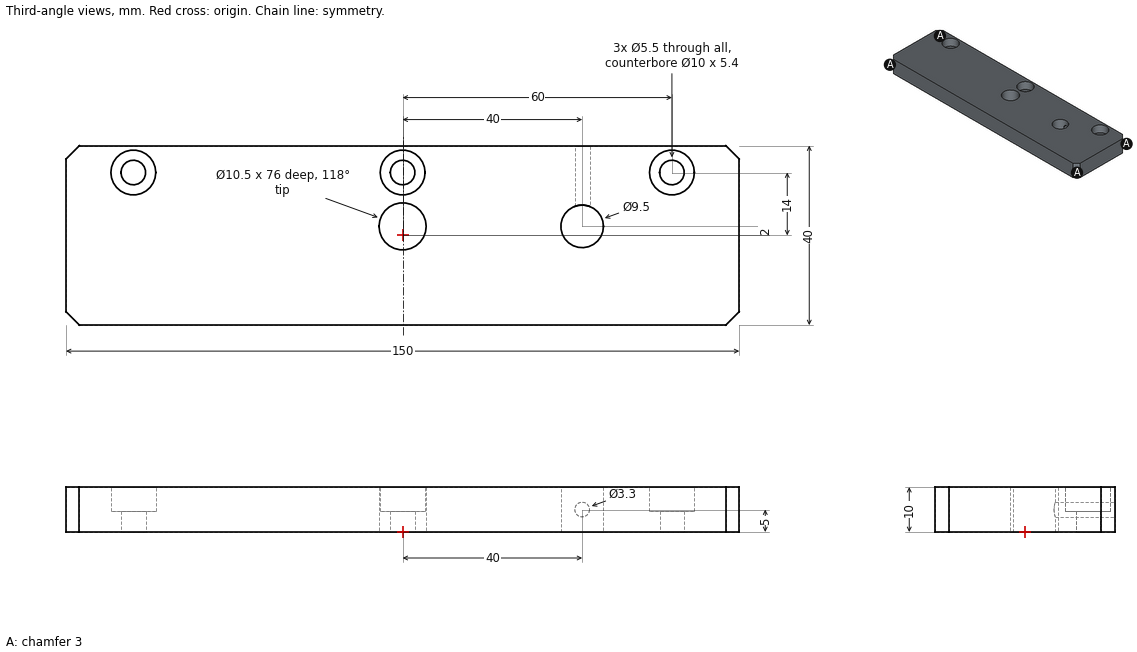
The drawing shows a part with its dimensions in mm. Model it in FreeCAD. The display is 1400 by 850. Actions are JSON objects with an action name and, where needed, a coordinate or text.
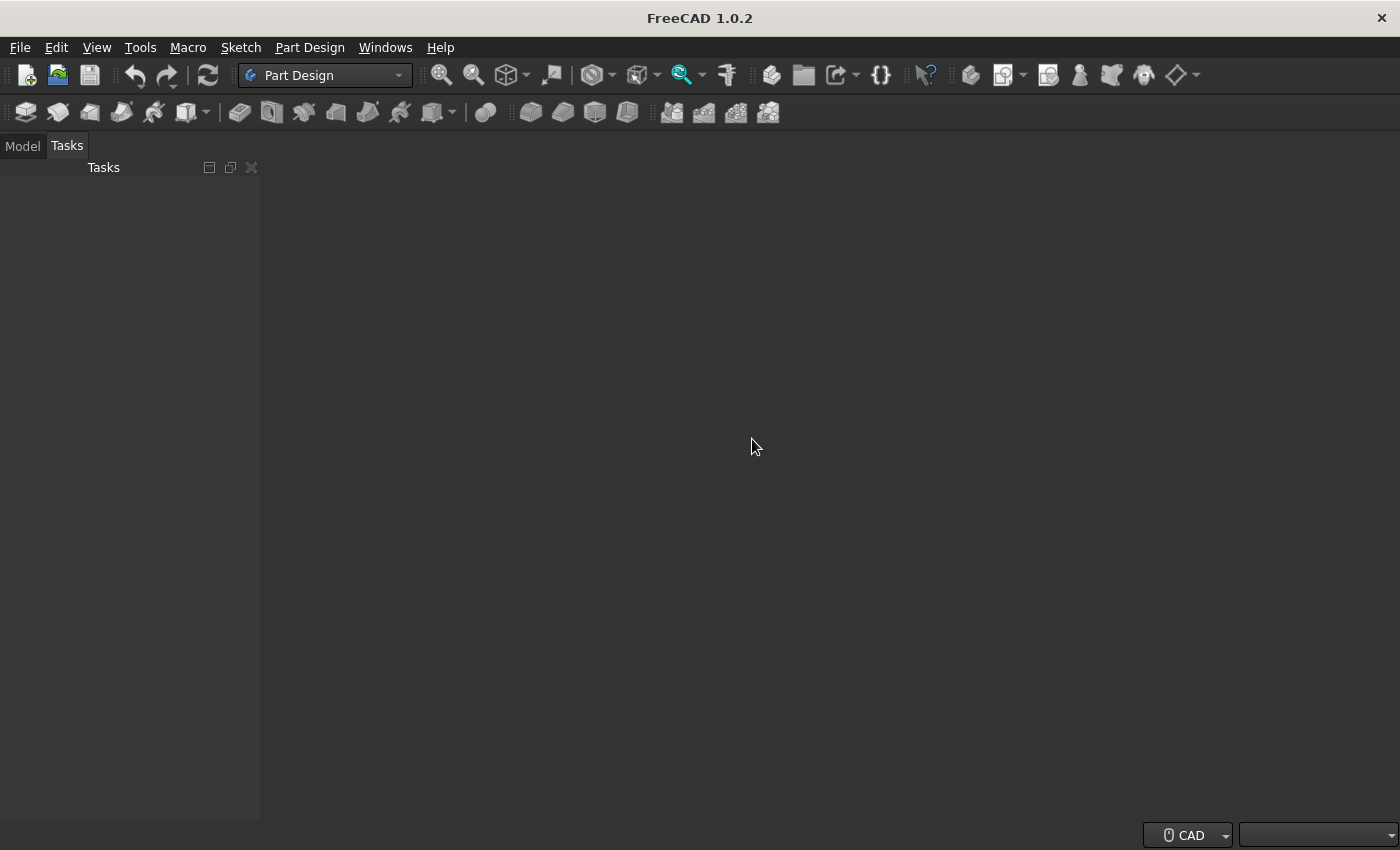
{"action": "left_click", "coordinate": [26, 76]}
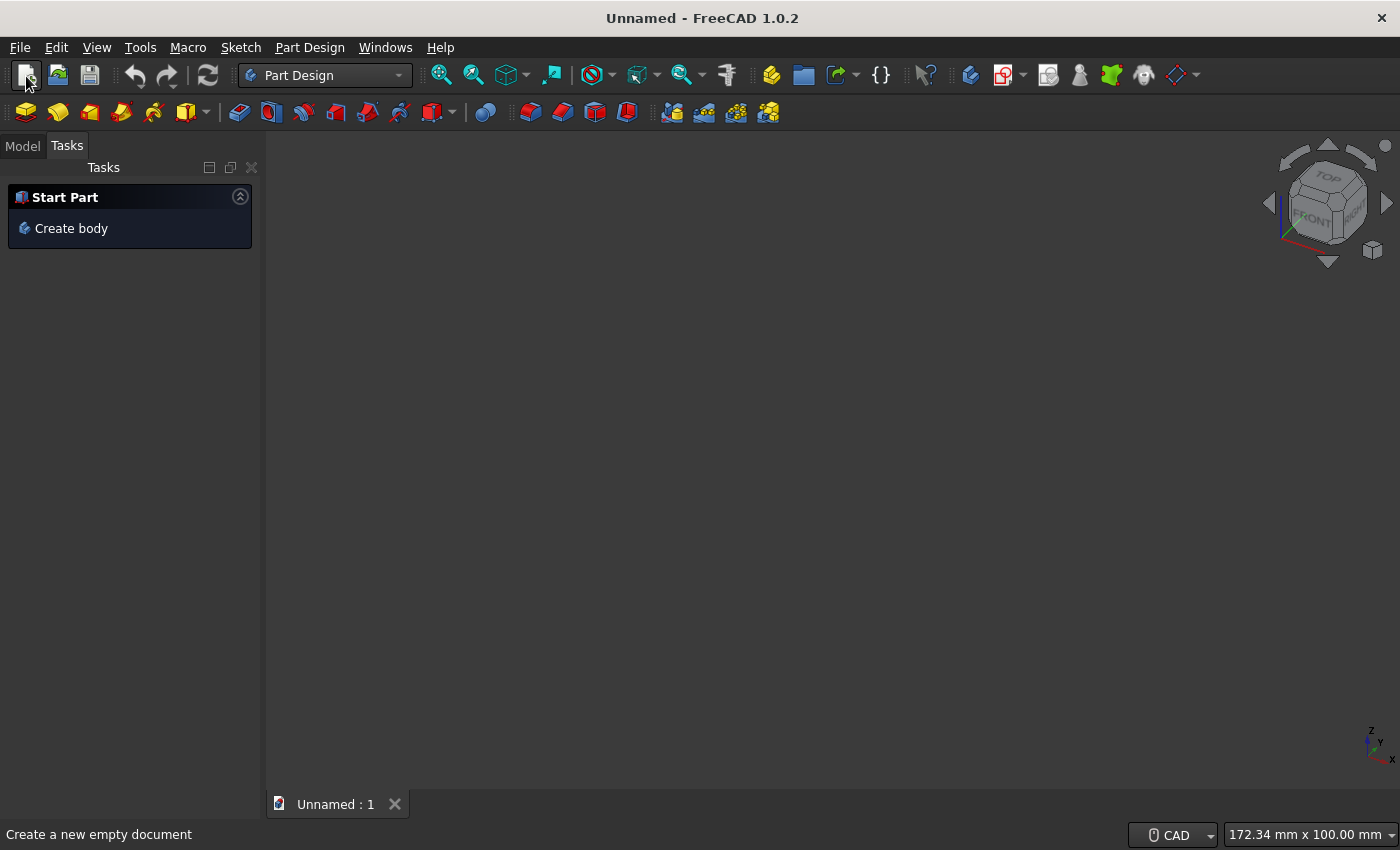
{"action": "left_click", "coordinate": [1004, 76]}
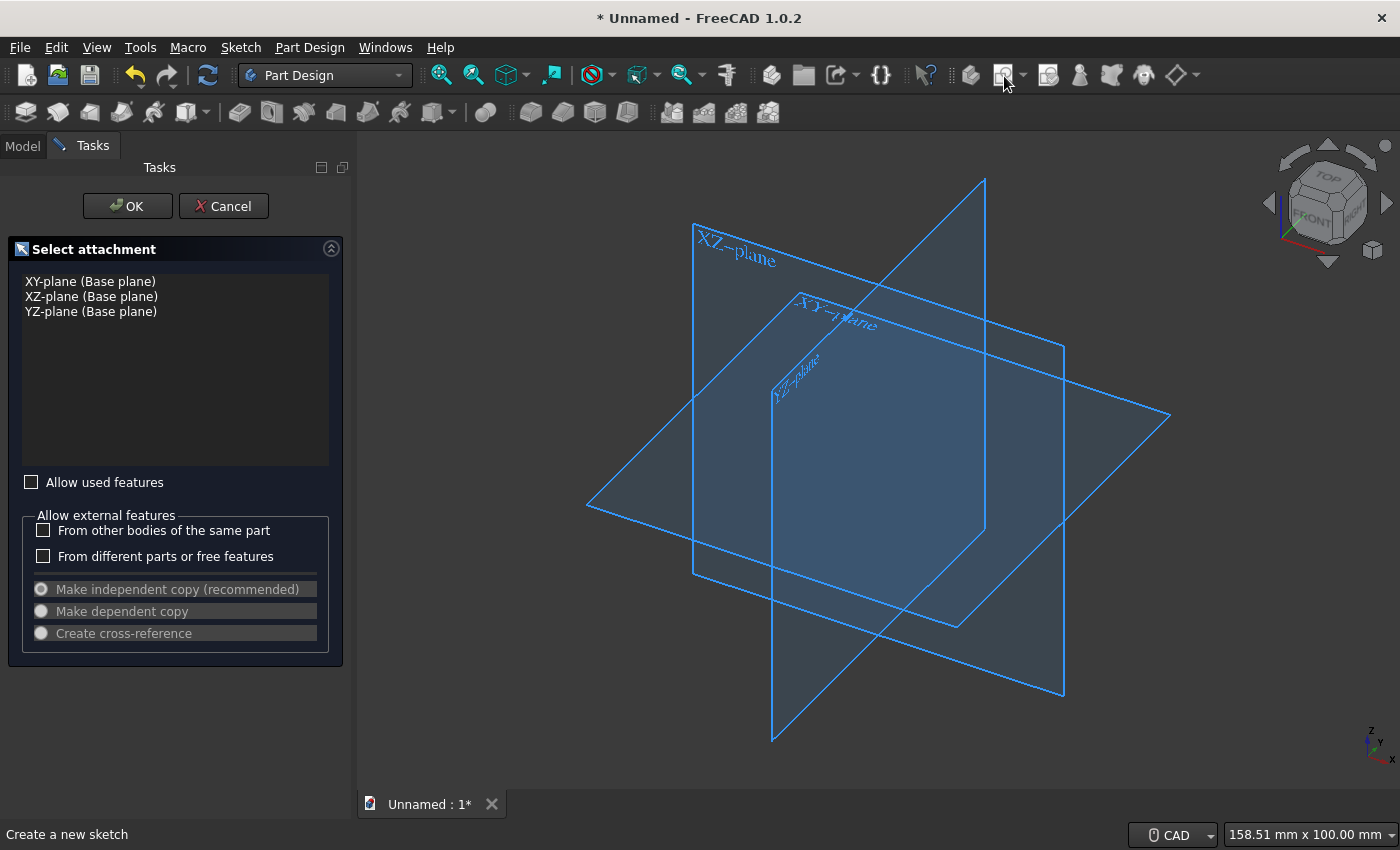
{"action": "left_click", "coordinate": [82, 282]}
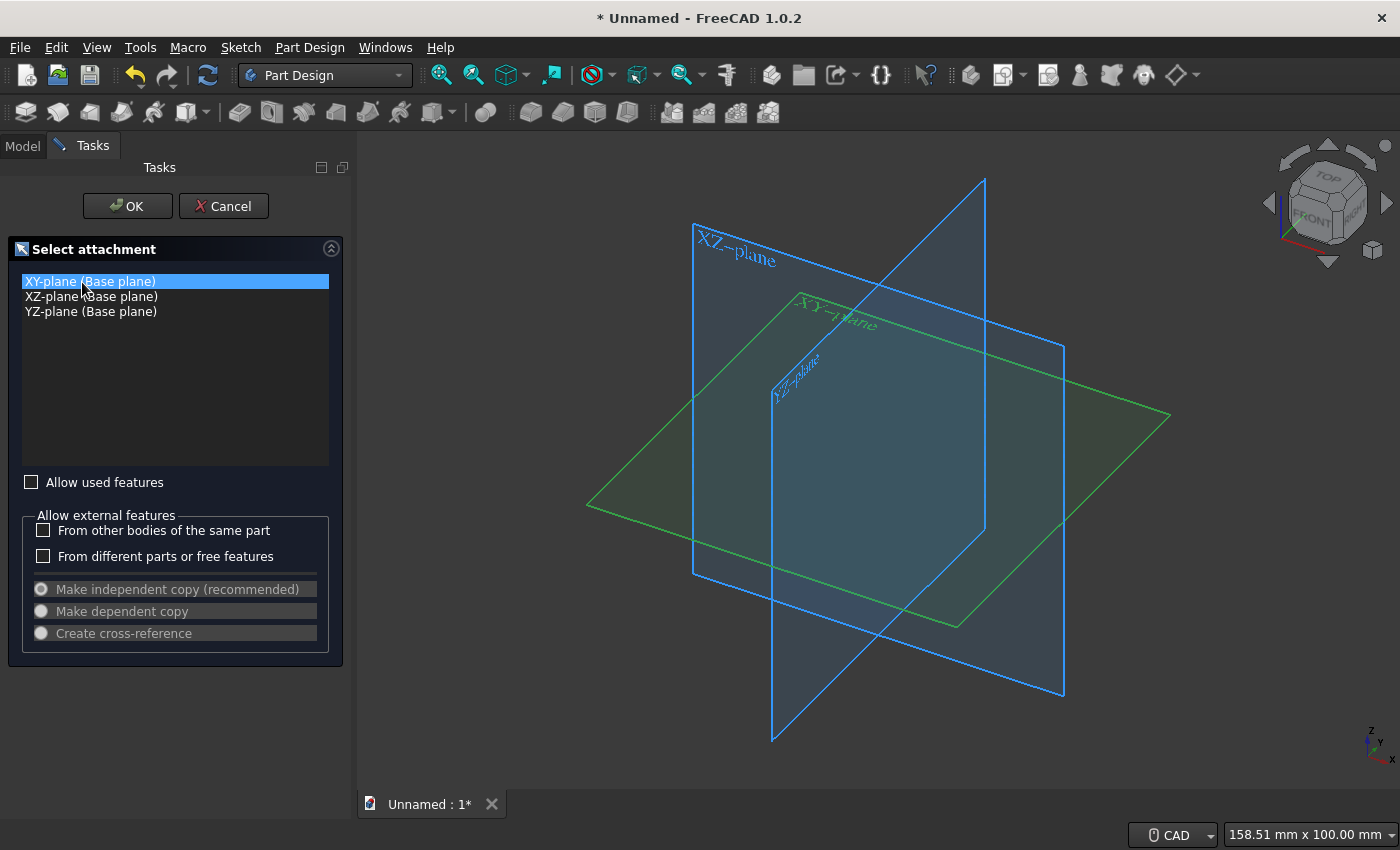
{"action": "left_click", "coordinate": [128, 206]}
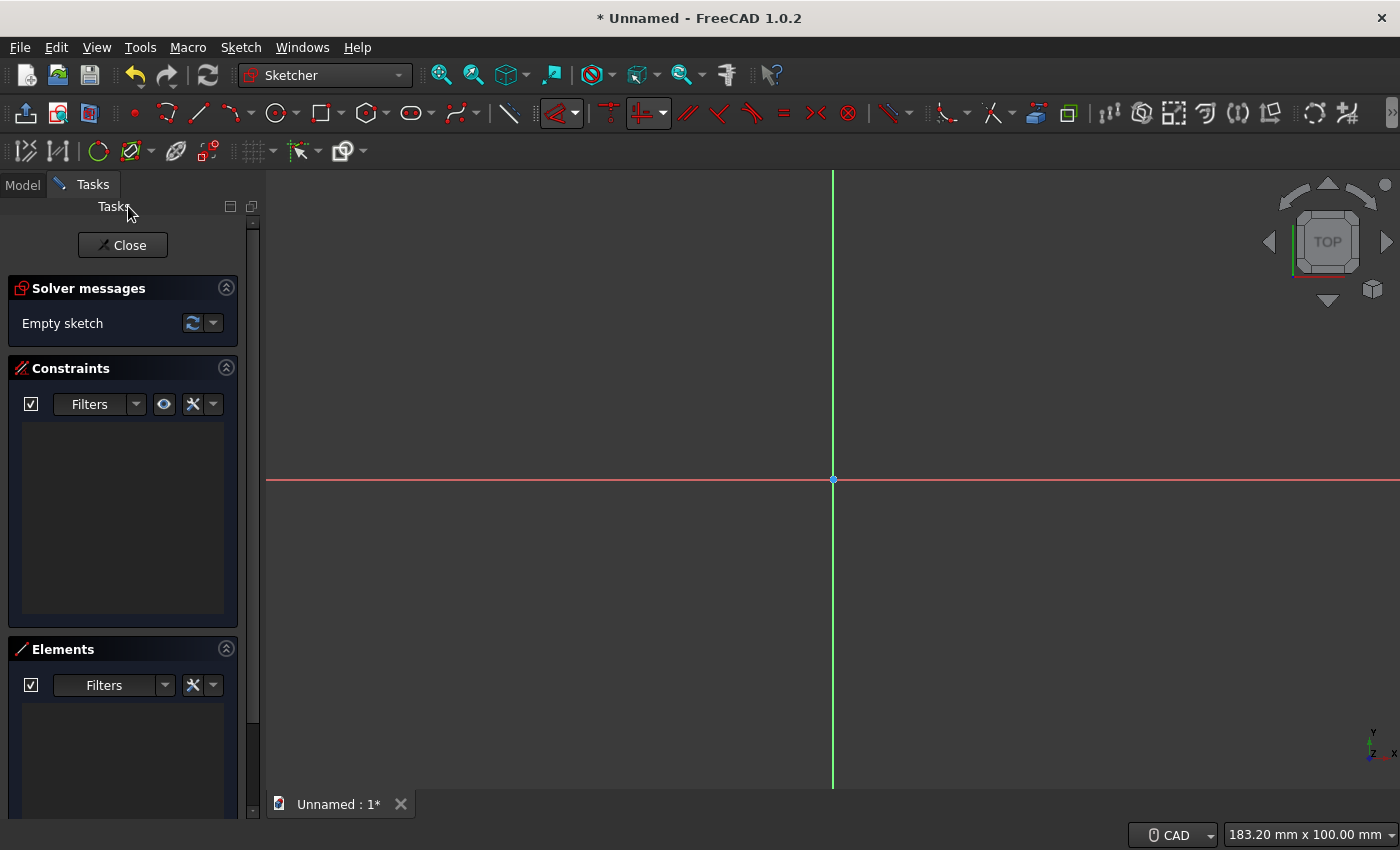
{"action": "scroll", "coordinate": [625, 480], "scroll_direction": "down", "scroll_amount": 2}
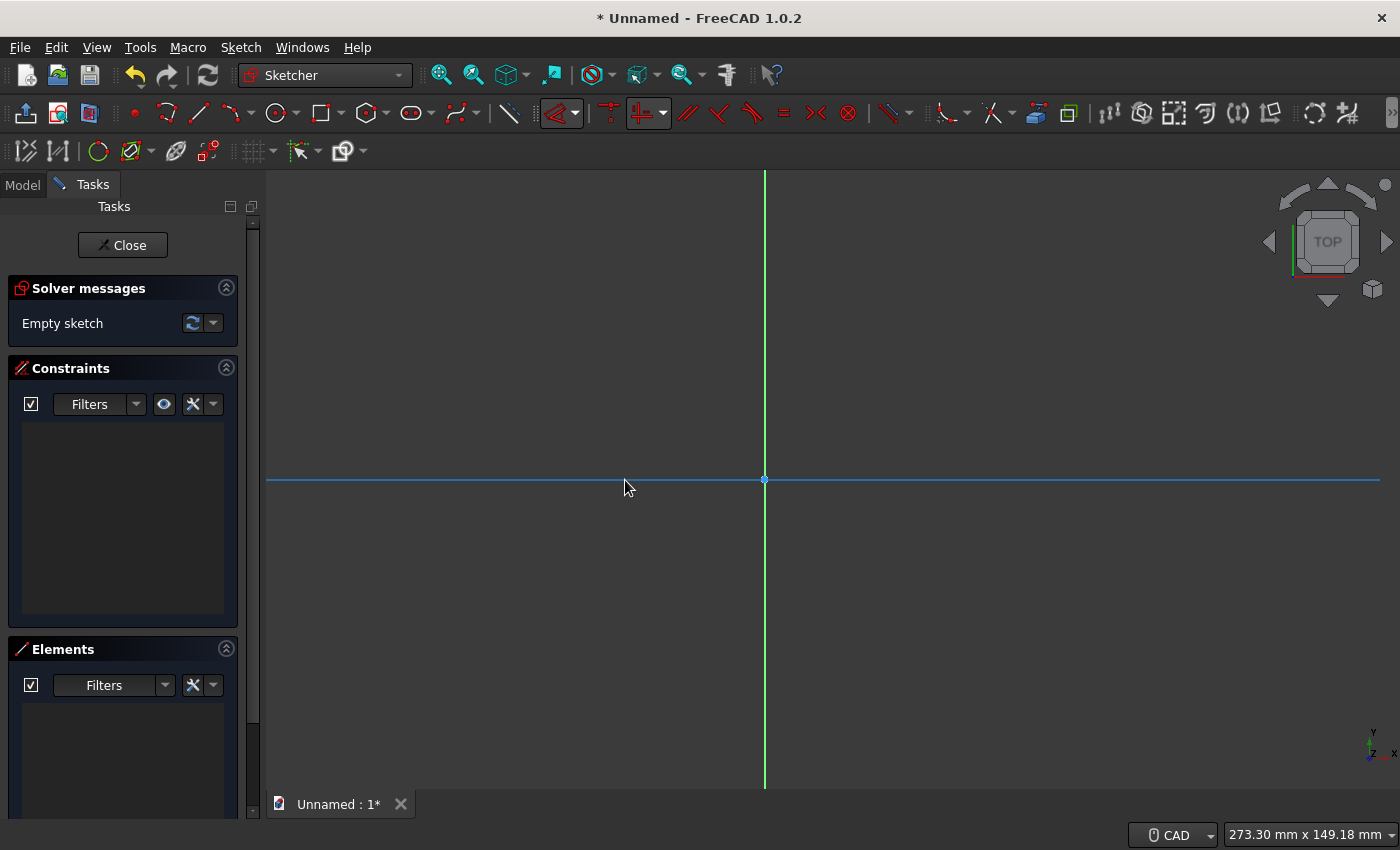
{"action": "key", "text": "g v"}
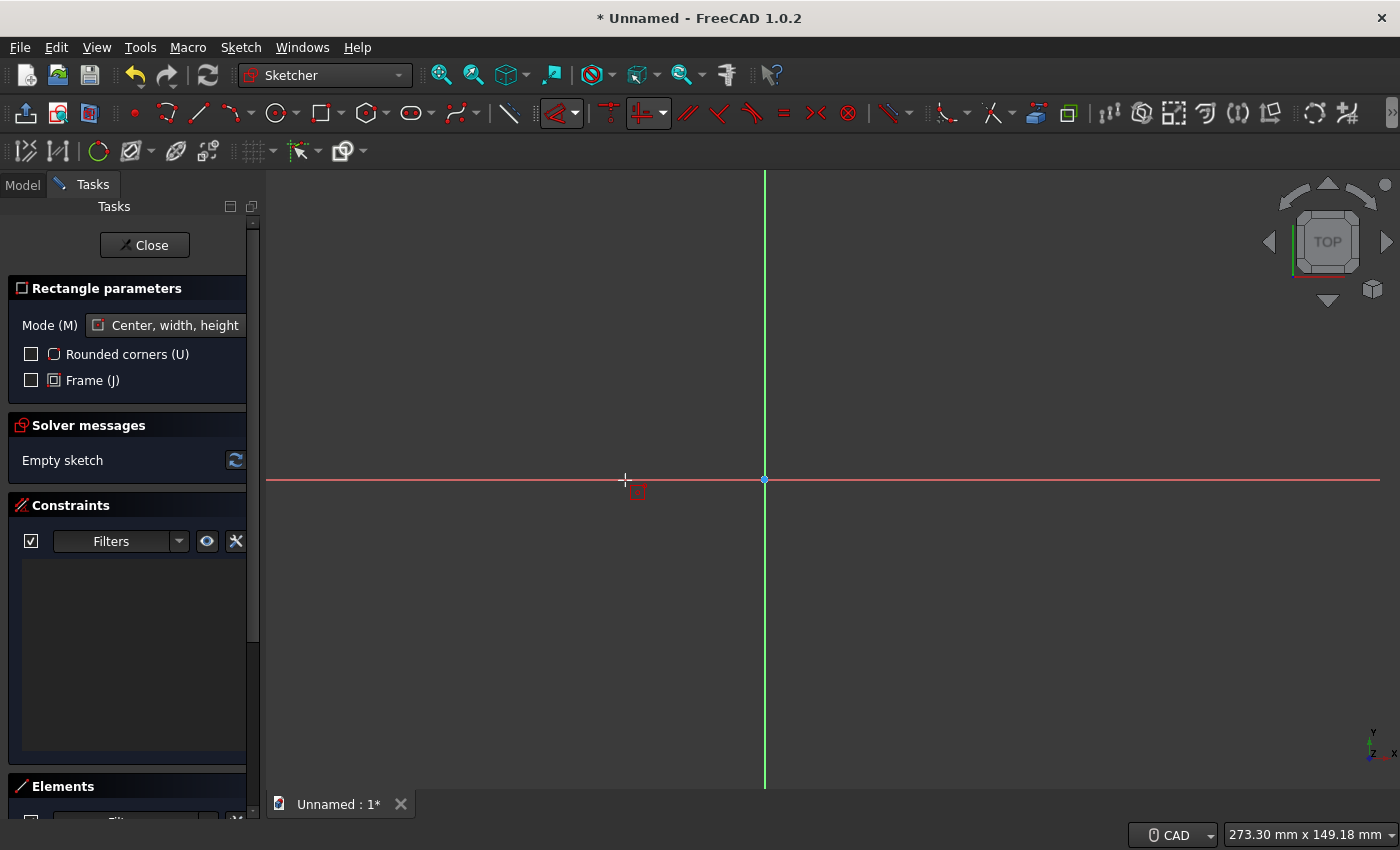
{"action": "left_click", "coordinate": [765, 480]}
{"action": "mouse_move", "coordinate": [1076, 397]}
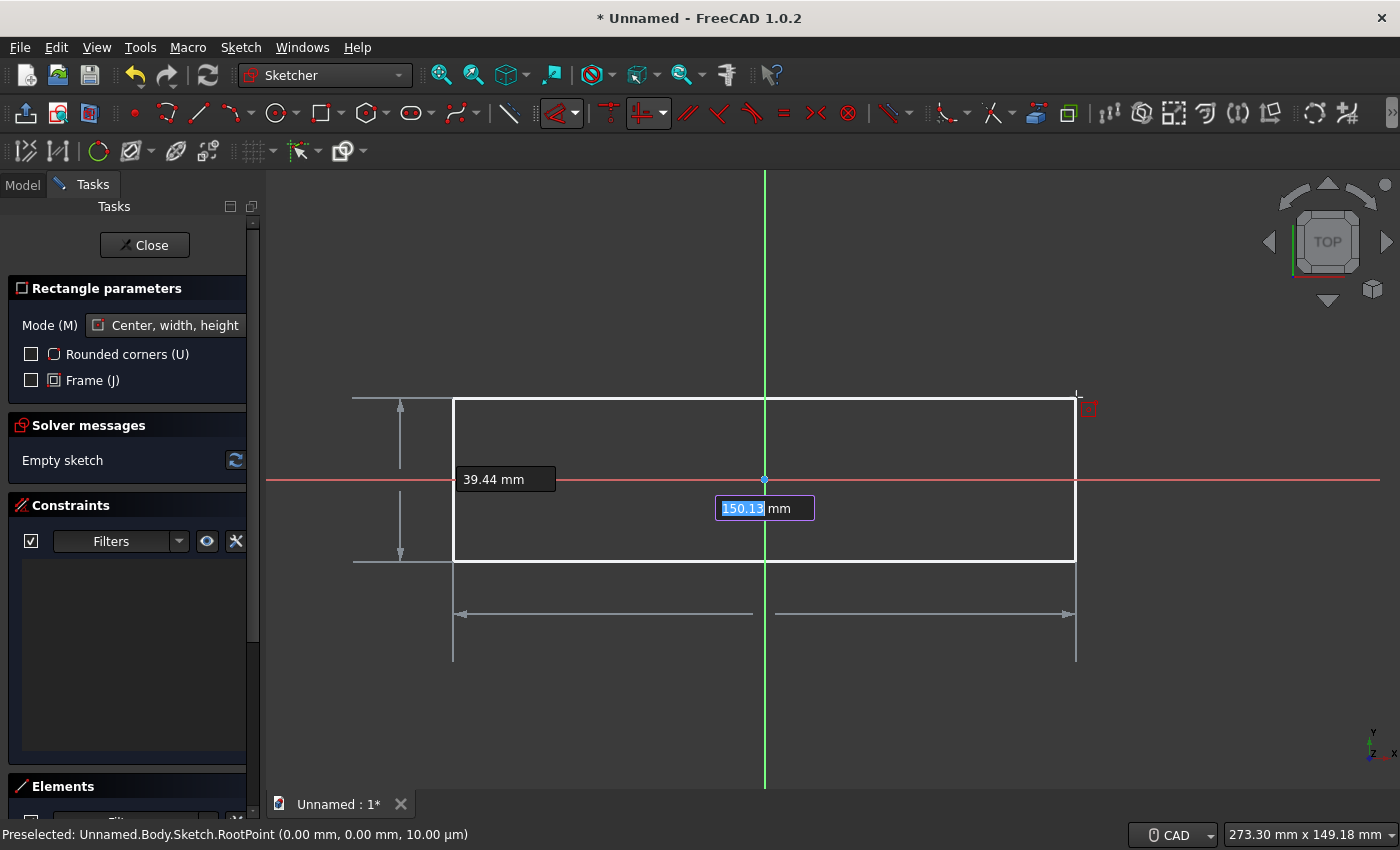
{"action": "type", "text": "150"}
{"action": "key", "text": "Tab"}
{"action": "type", "text": "40"}
{"action": "key", "text": "Return"}
{"action": "key", "text": "Escape"}